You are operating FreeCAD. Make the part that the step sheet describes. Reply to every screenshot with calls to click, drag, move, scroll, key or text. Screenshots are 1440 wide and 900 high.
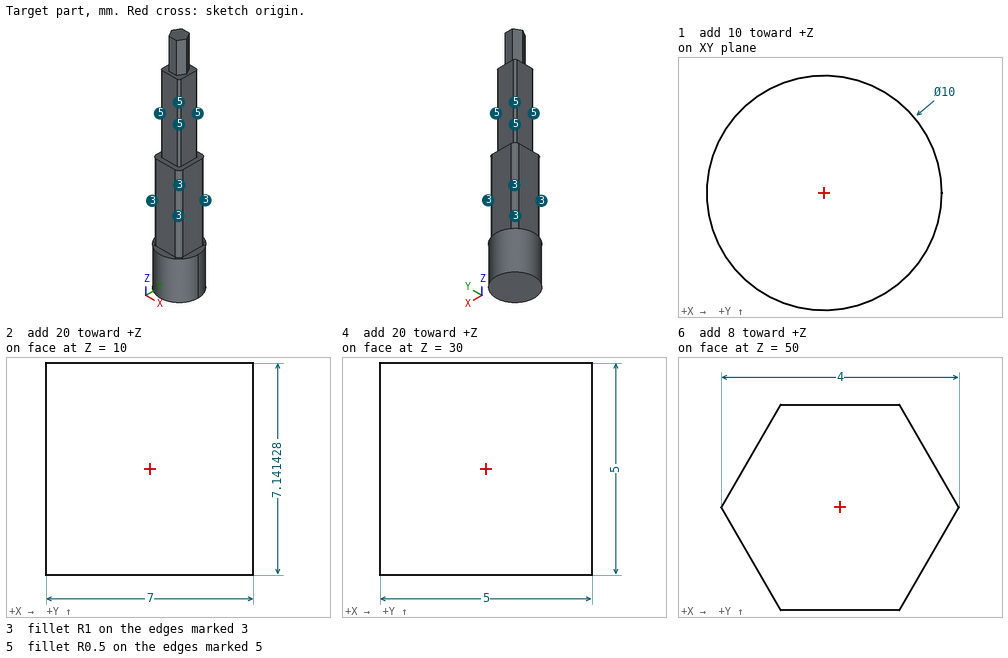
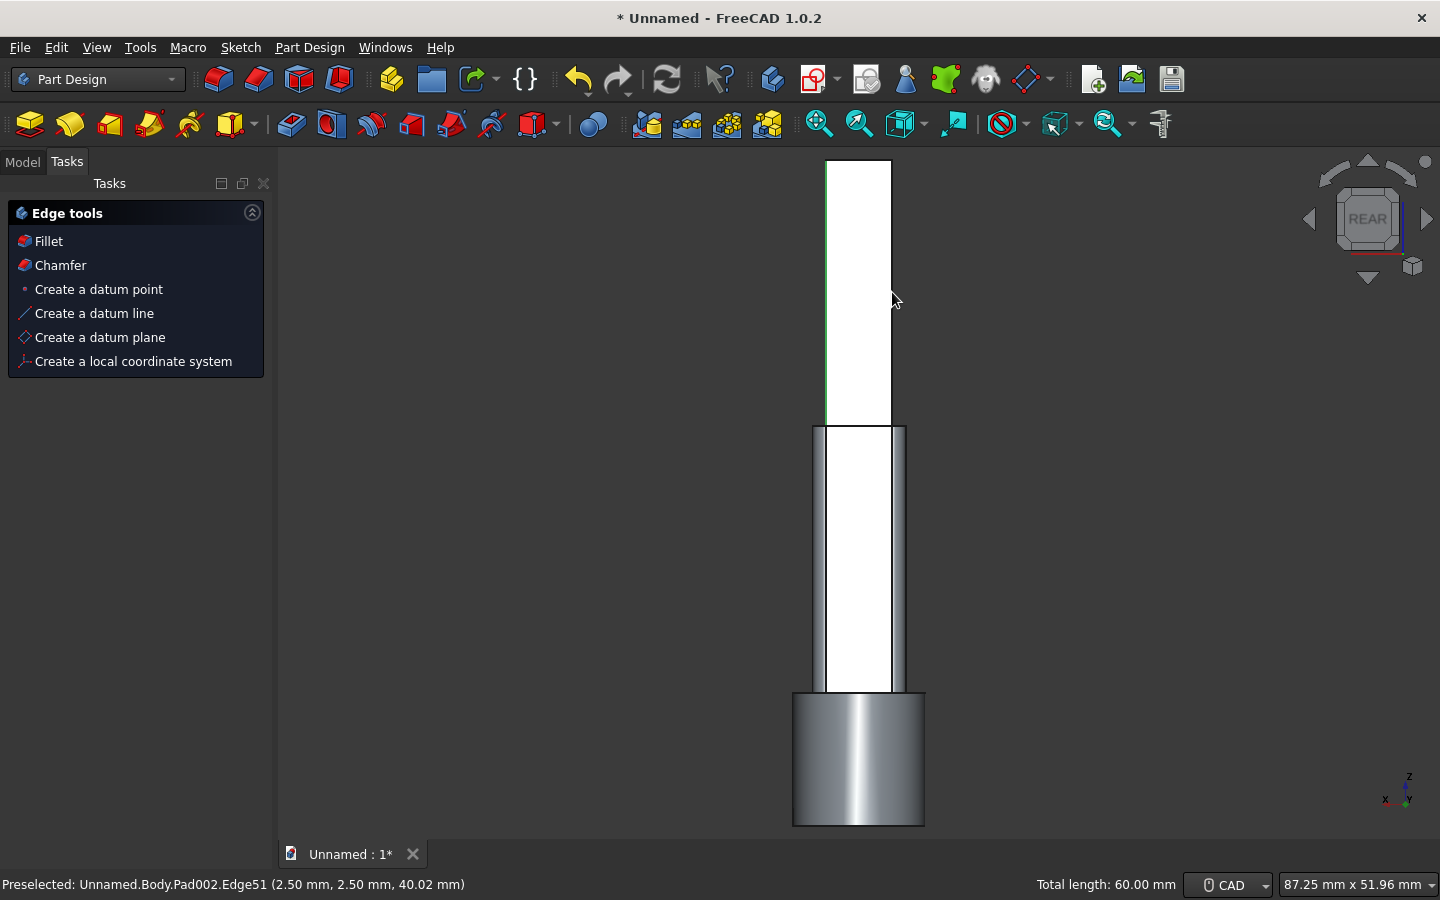
click(892, 292, ctrl)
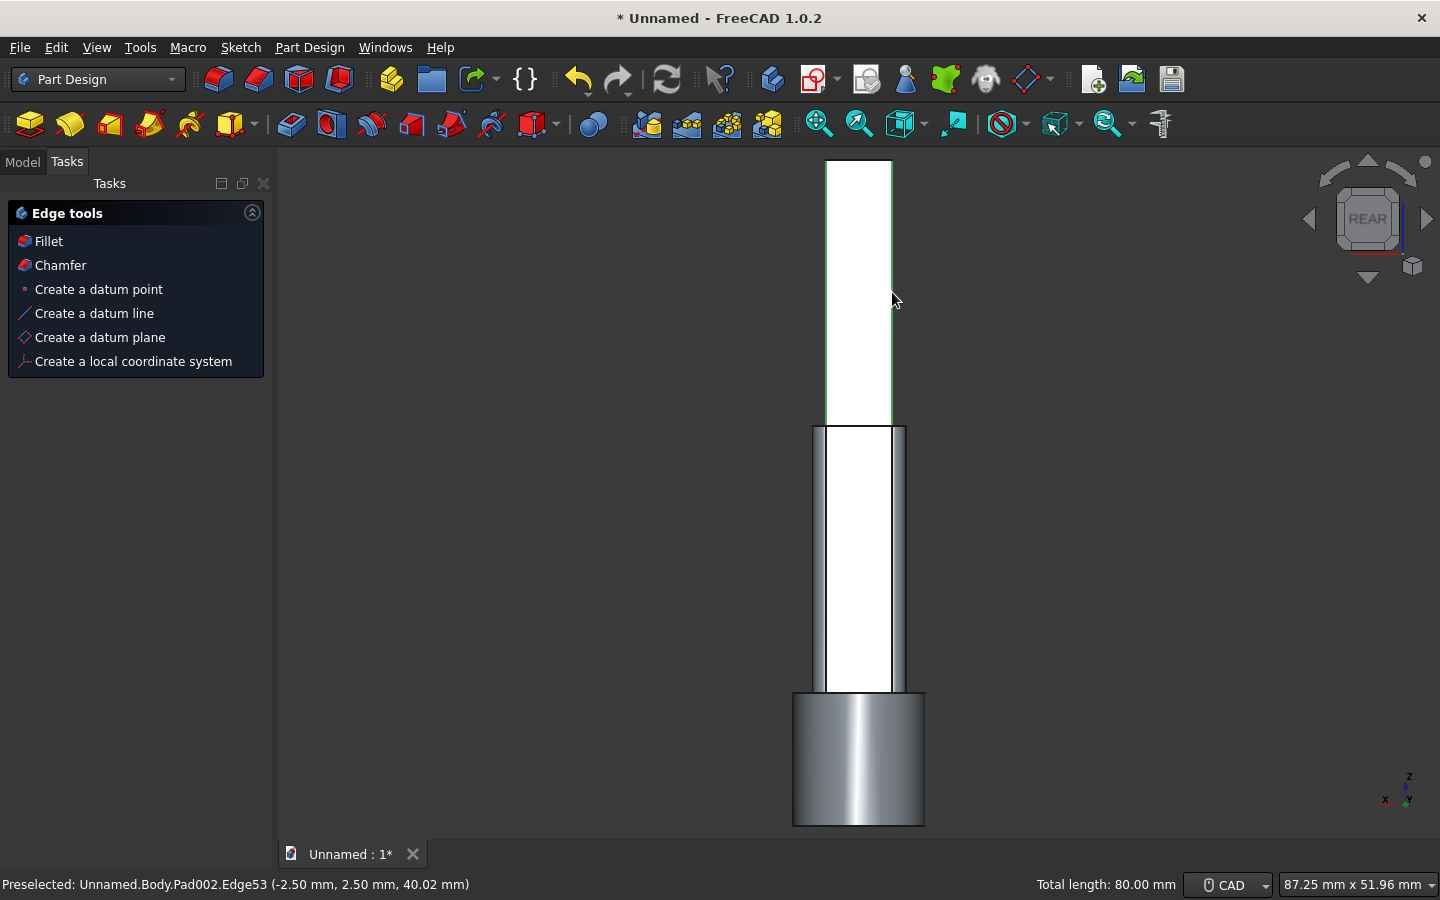
click(220, 80)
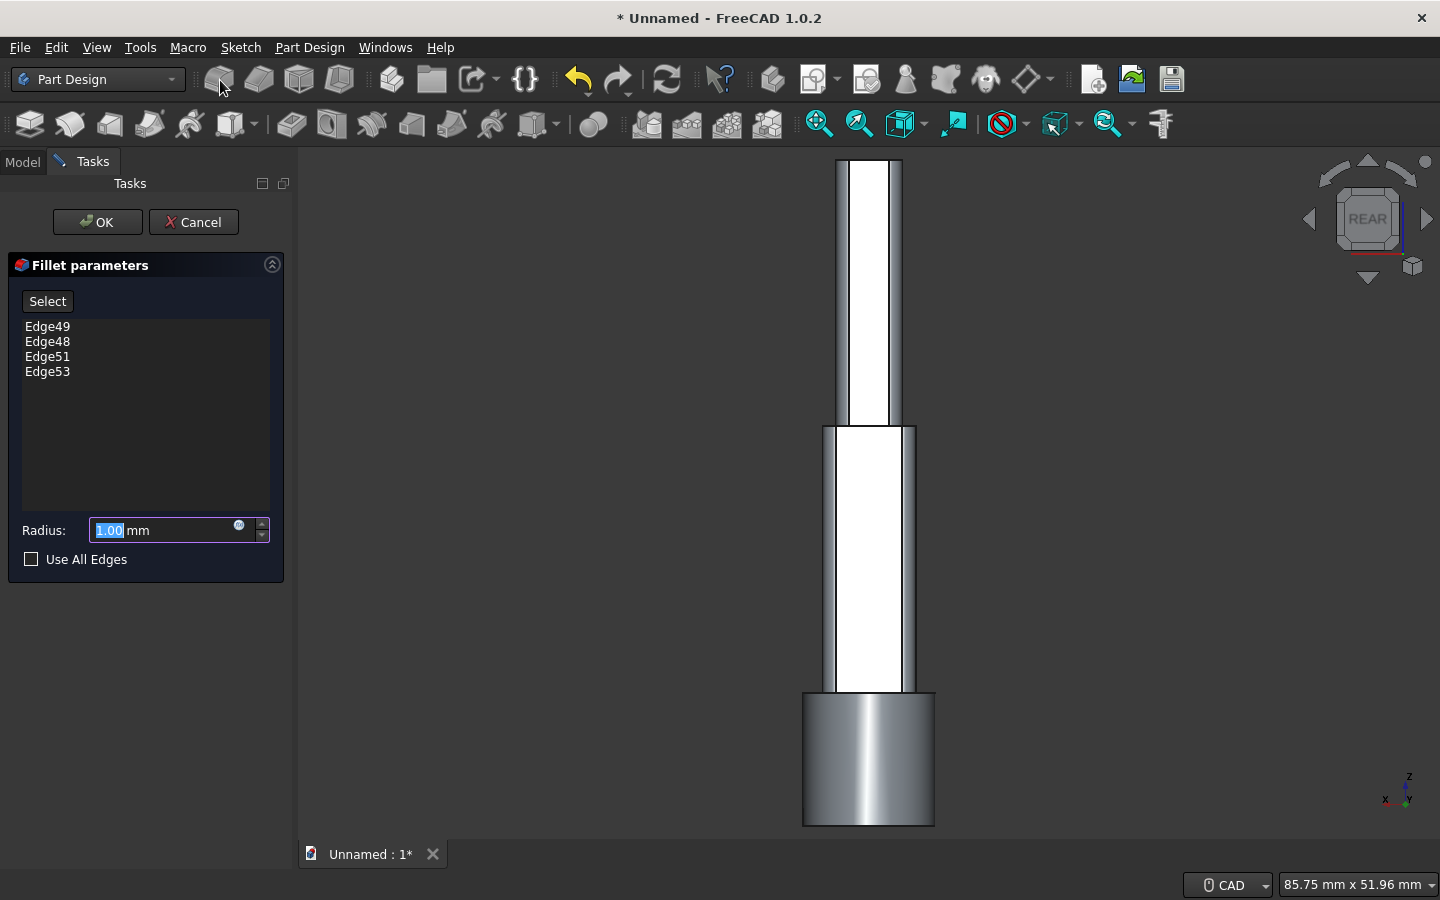
text(0.5)
key(Tab)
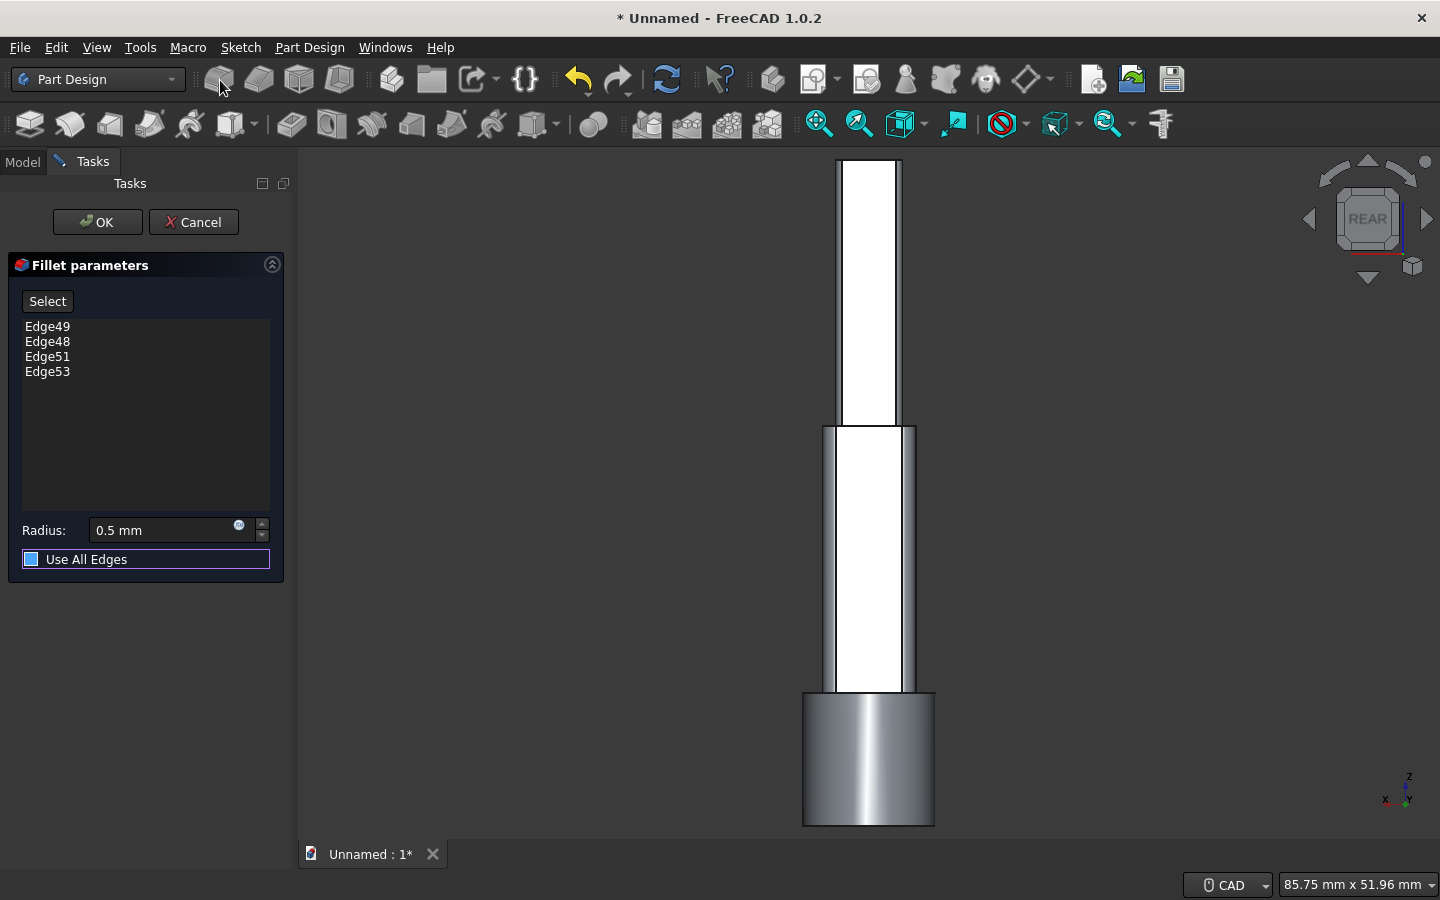
click(98, 222)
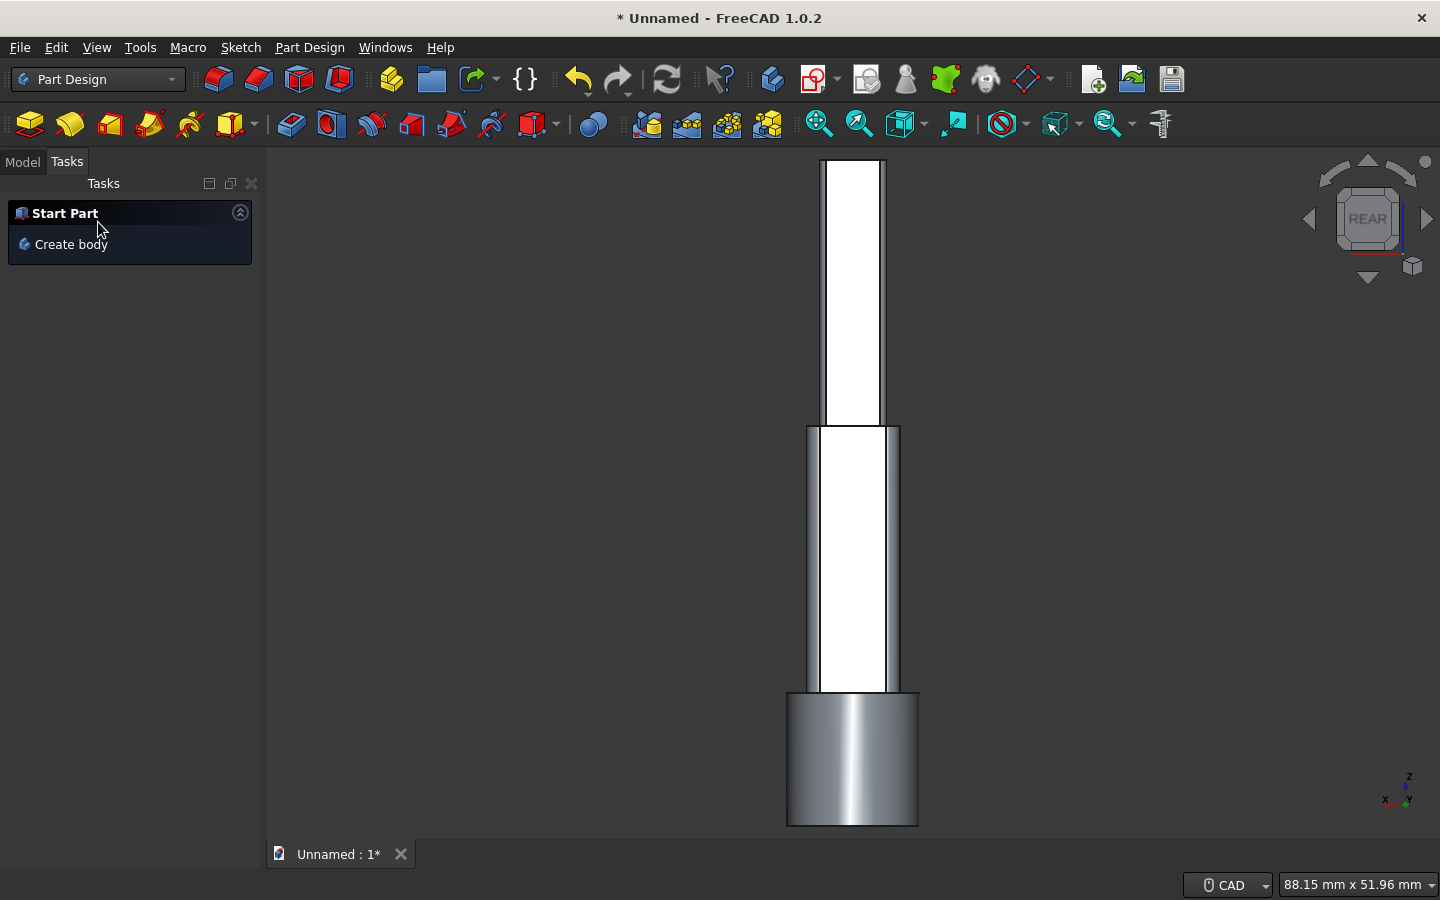
key(0)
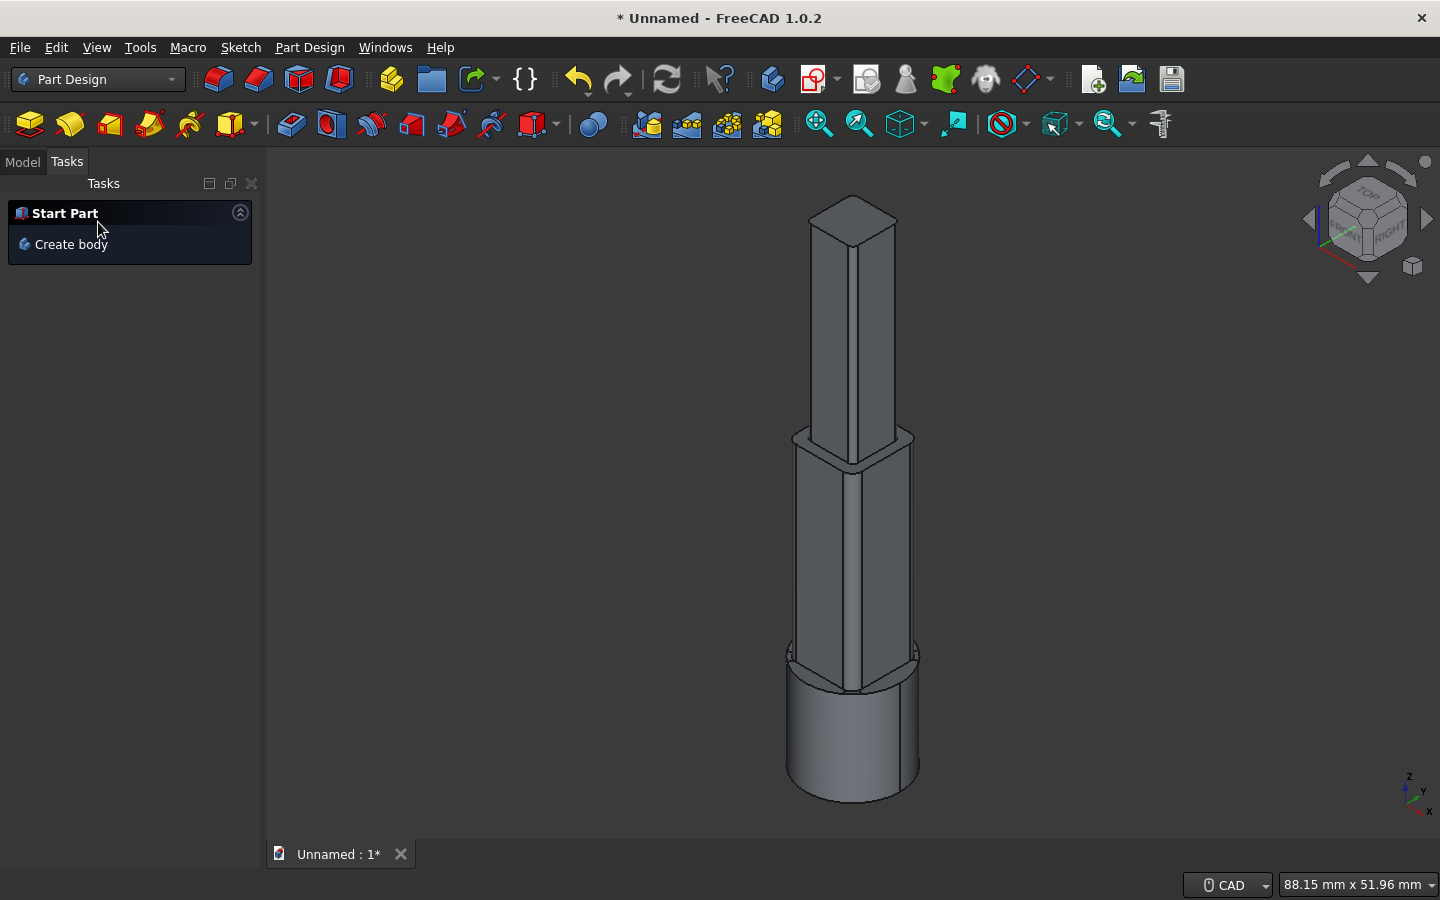
click(853, 220)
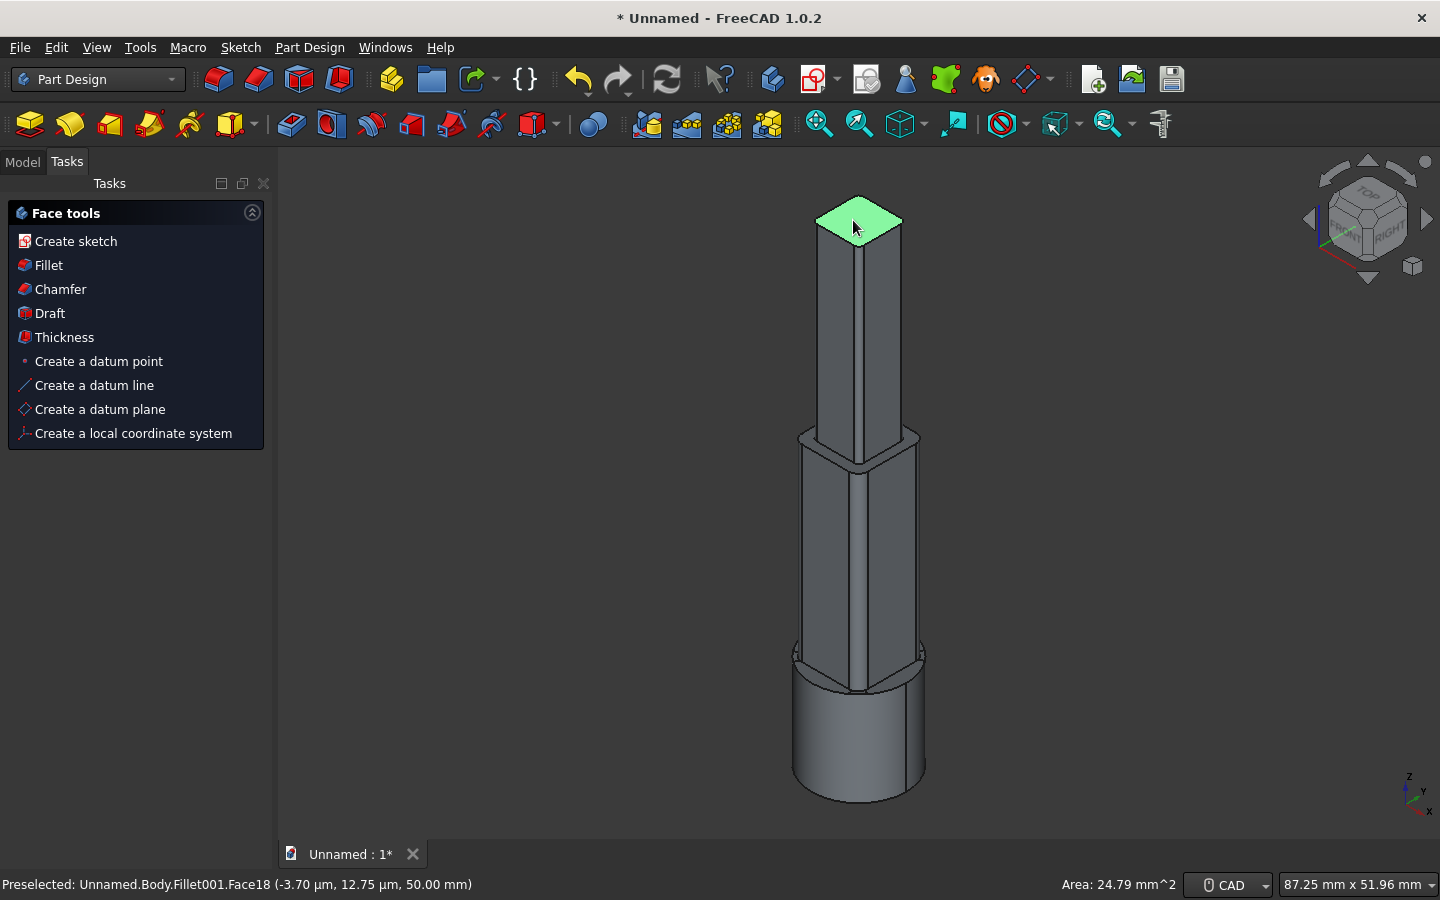
click(814, 80)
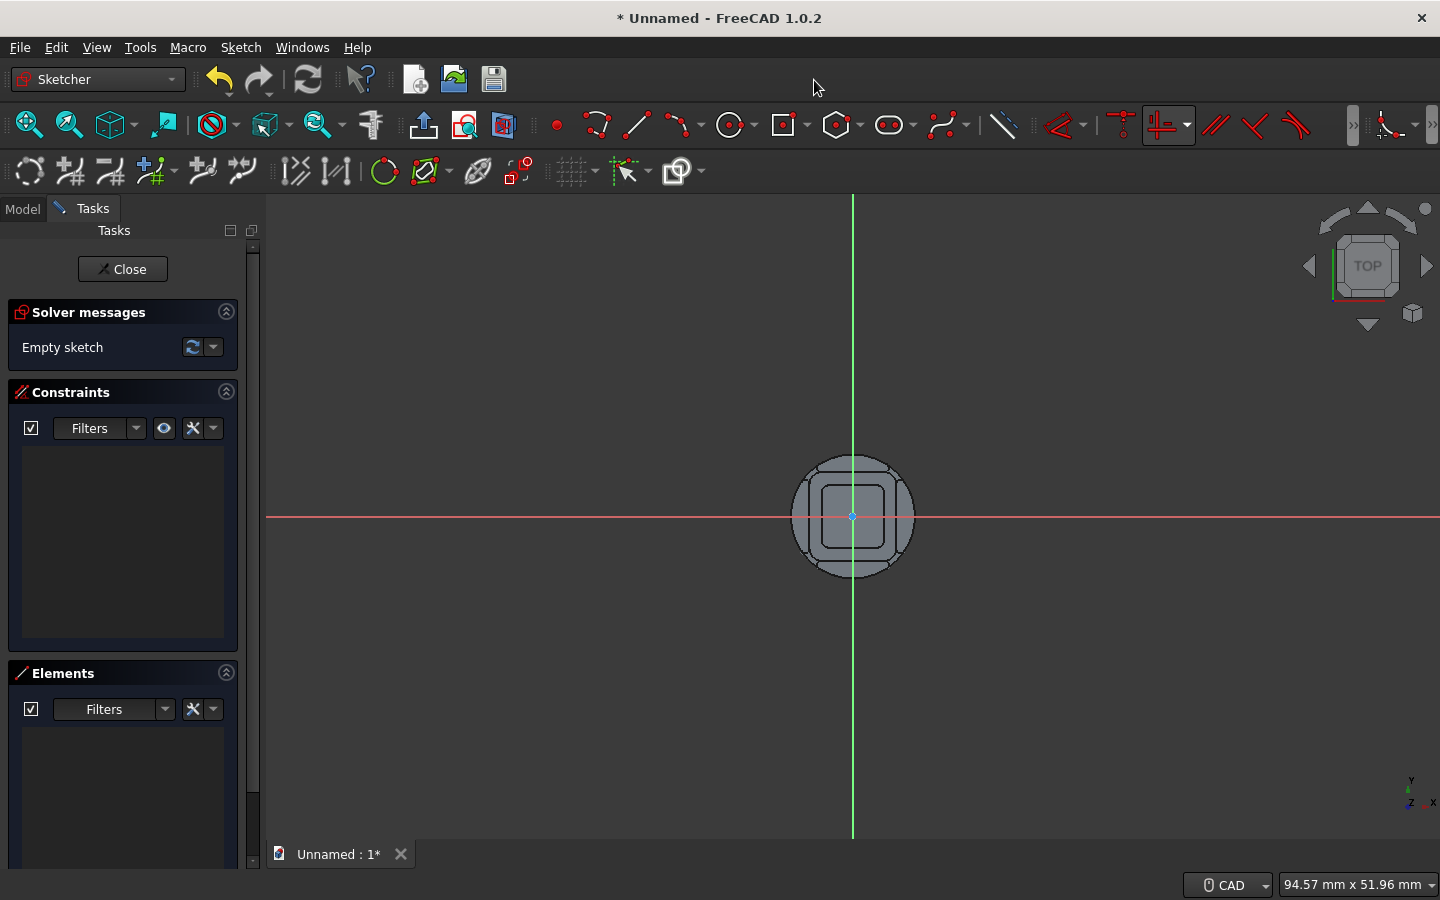
scroll(861, 517, up, 11)